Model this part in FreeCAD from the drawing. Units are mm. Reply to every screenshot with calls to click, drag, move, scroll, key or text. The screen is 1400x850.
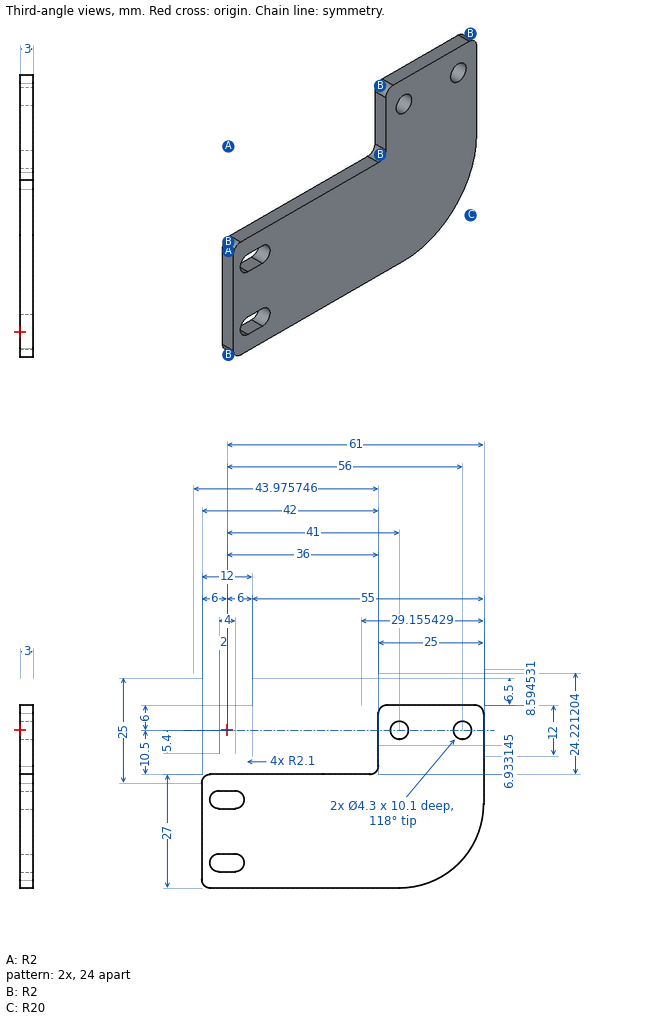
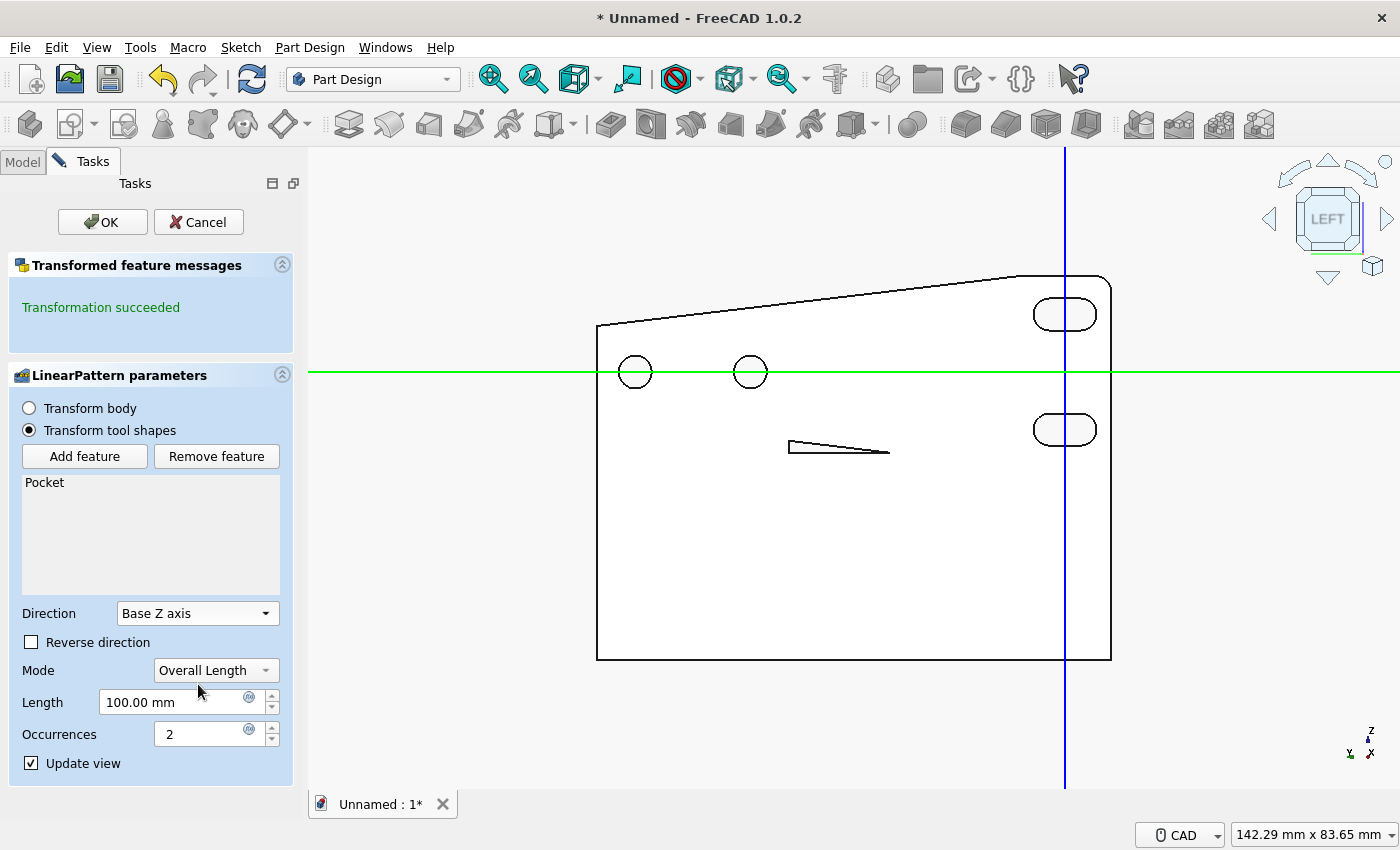
click(217, 670)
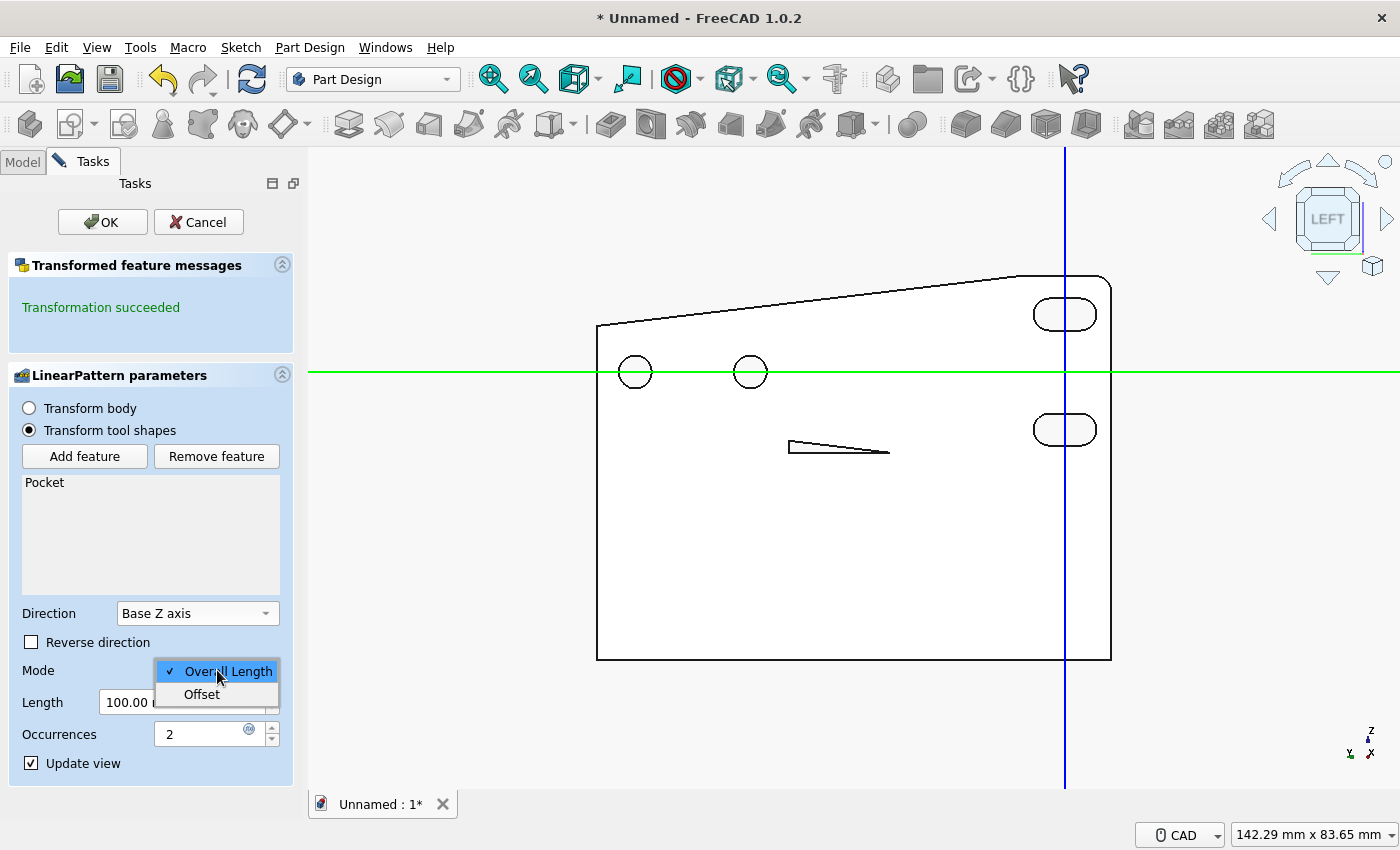
click(216, 694)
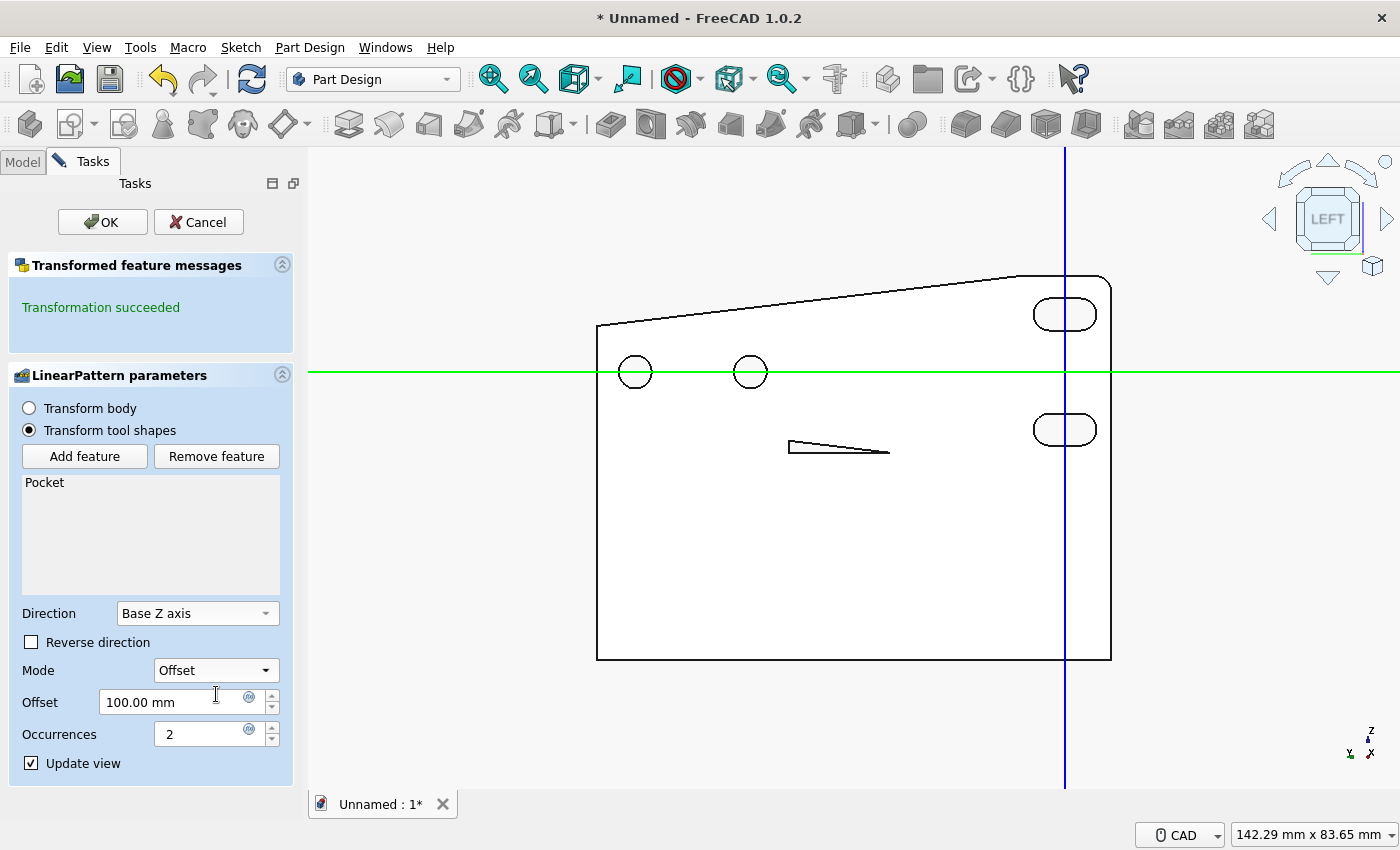
triple_click(182, 702)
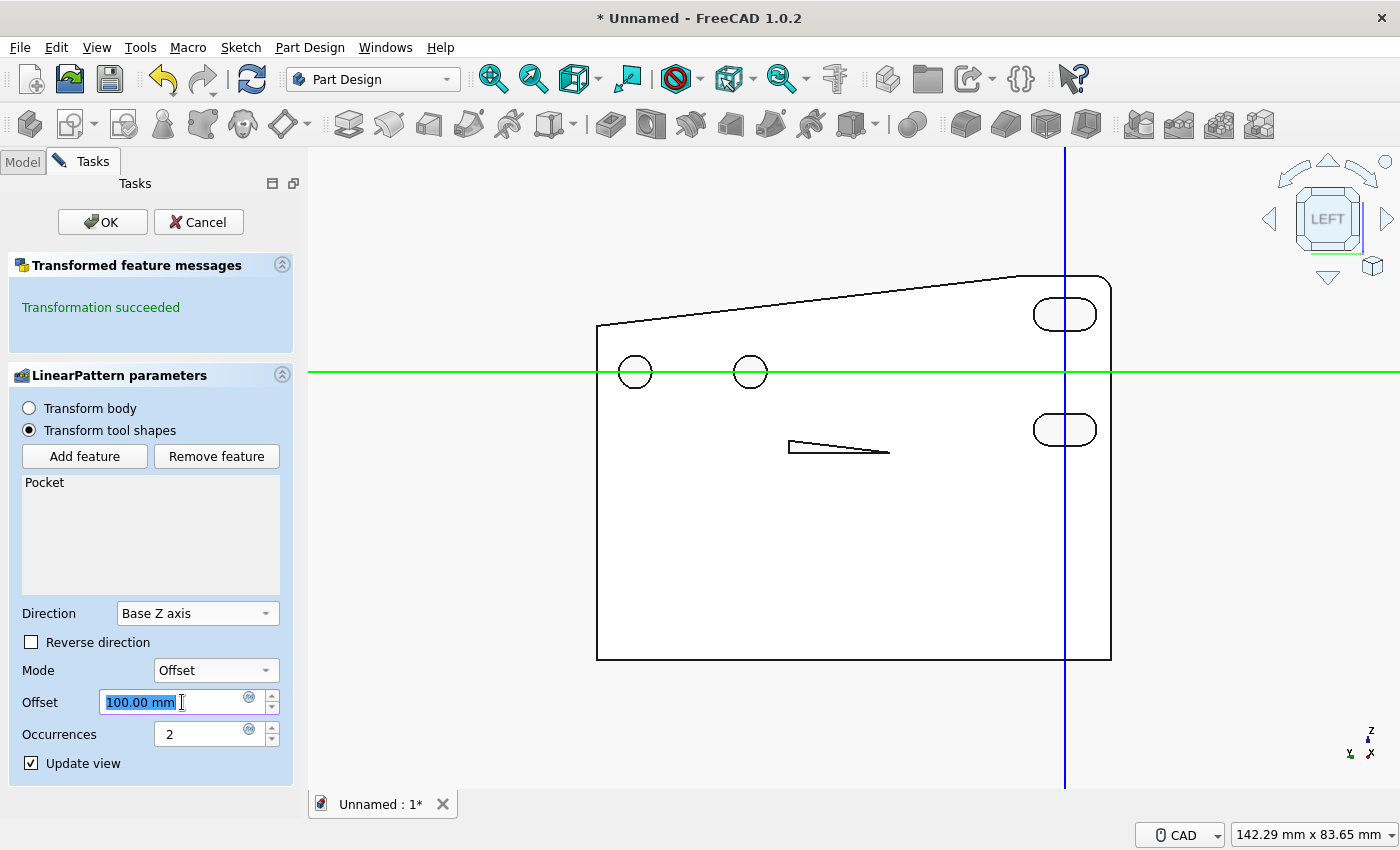
text(24)
key(Tab)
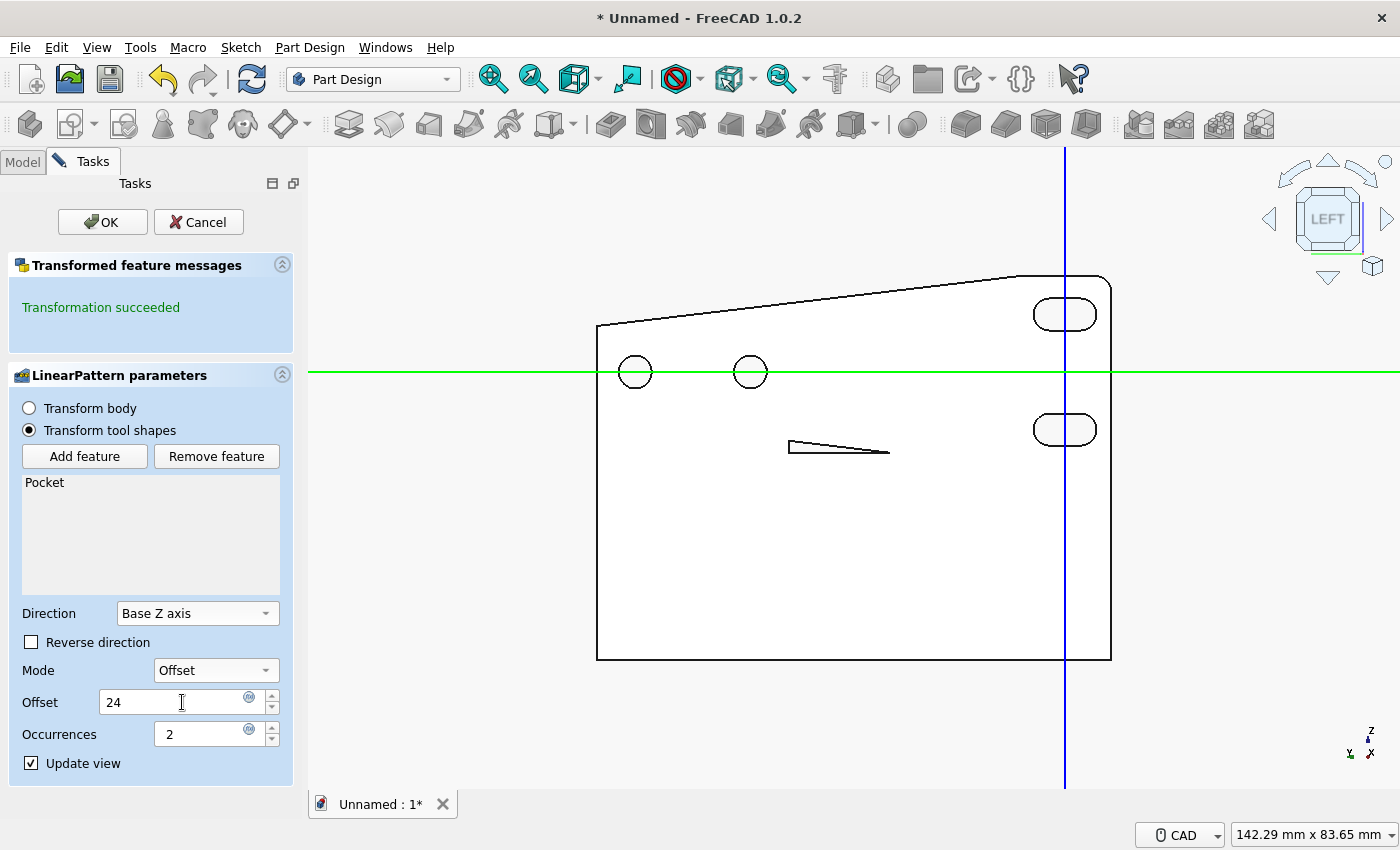
triple_click(209, 734)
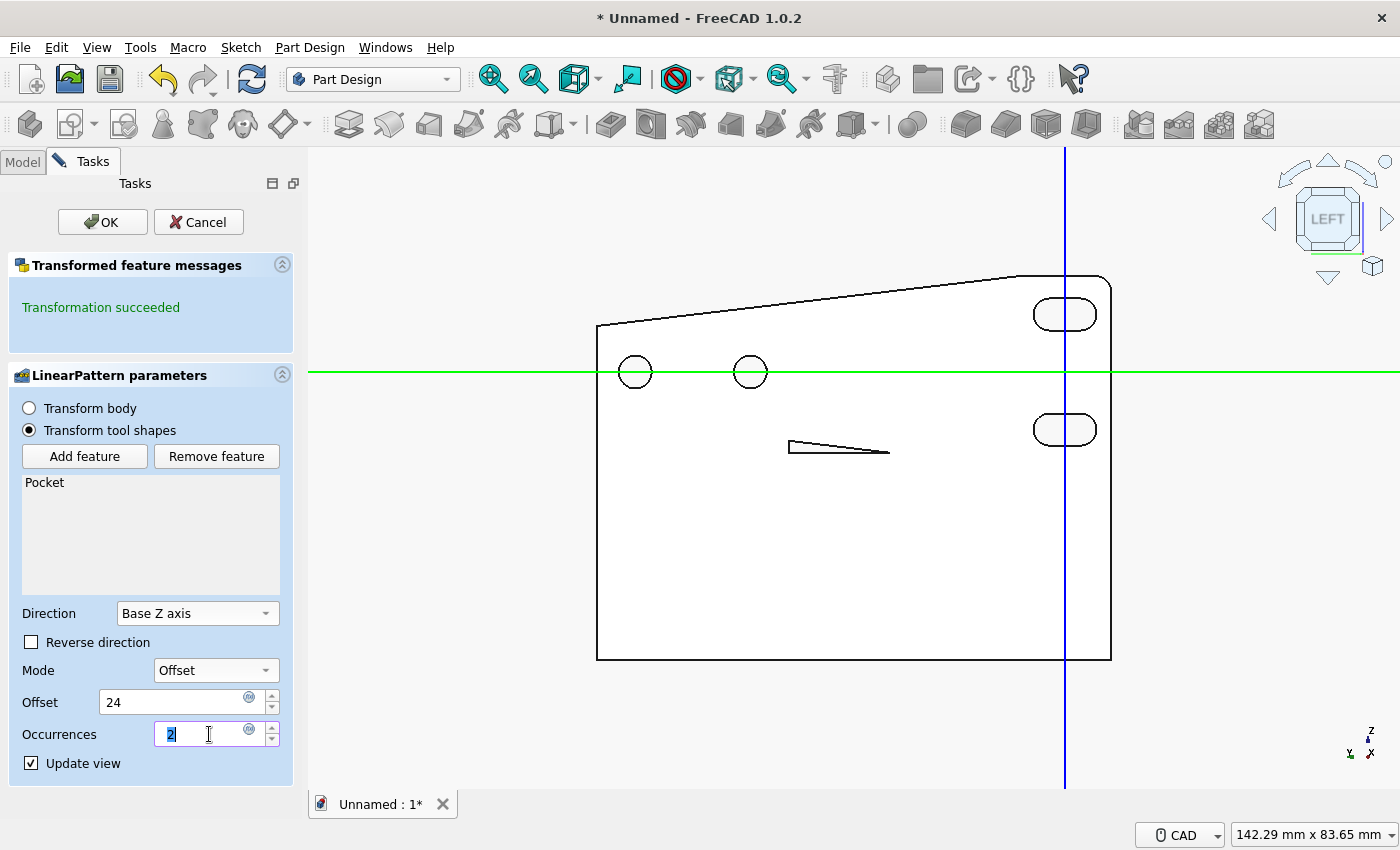
text(2)
key(Tab)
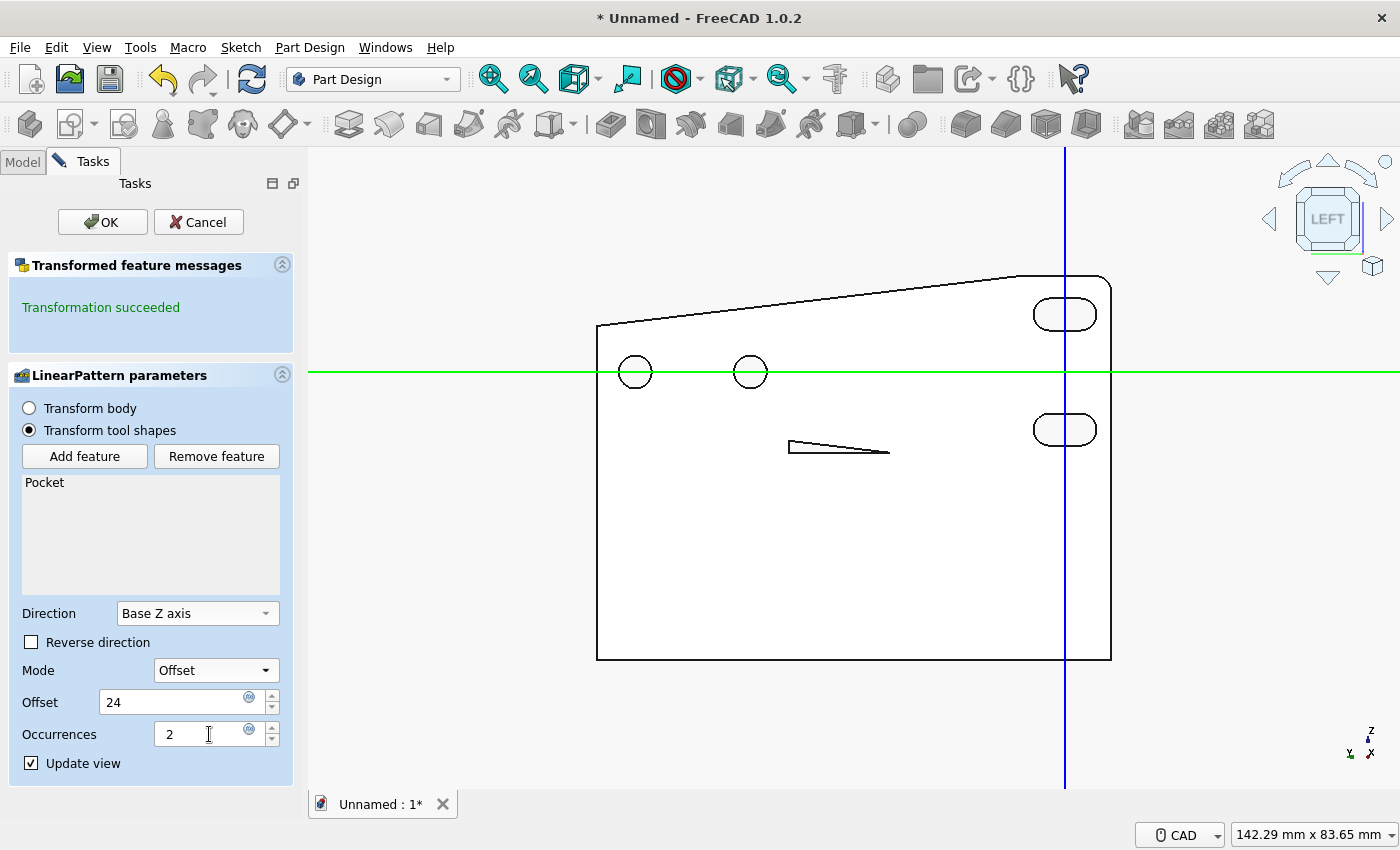
click(30, 642)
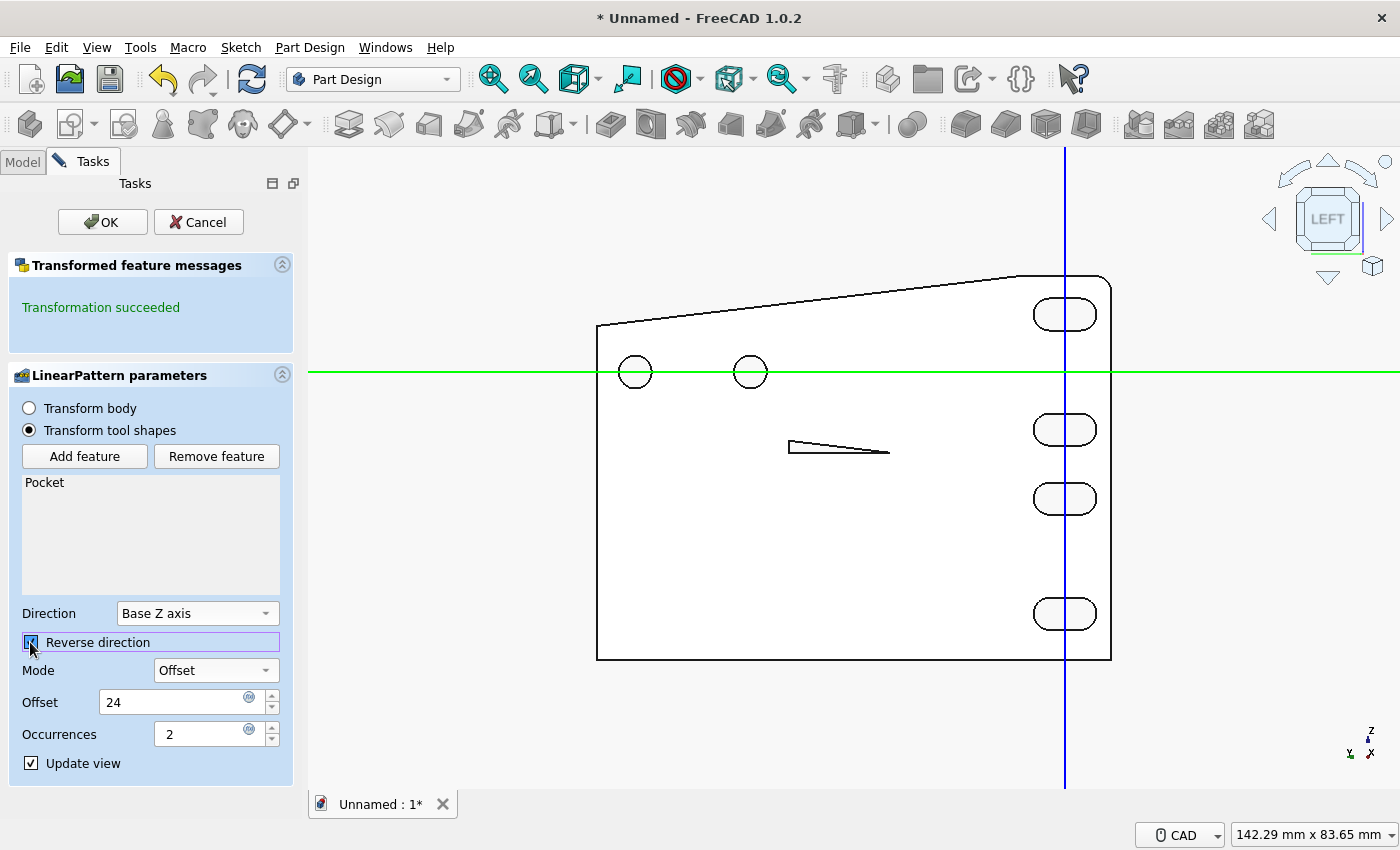
click(103, 222)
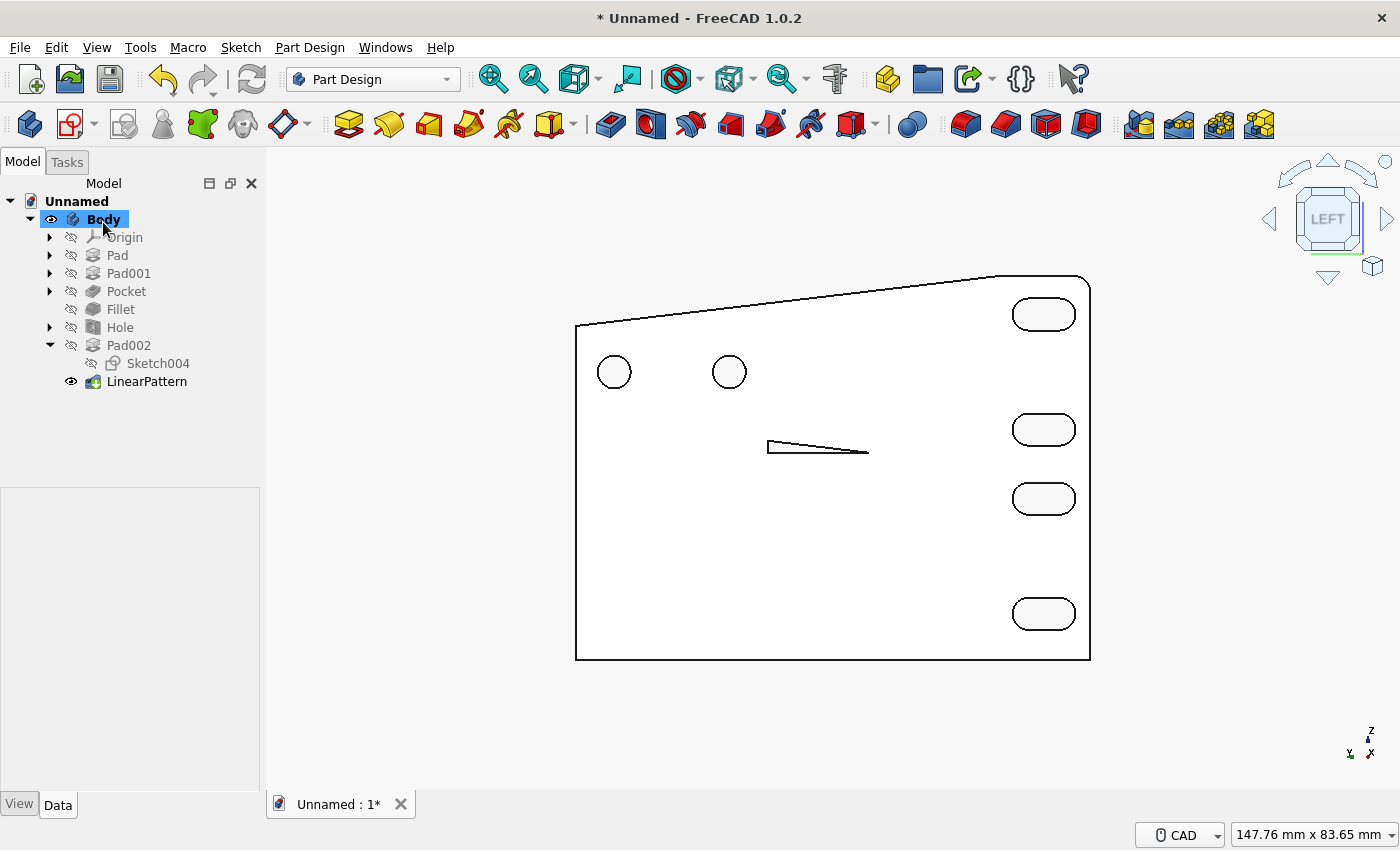
click(686, 522)